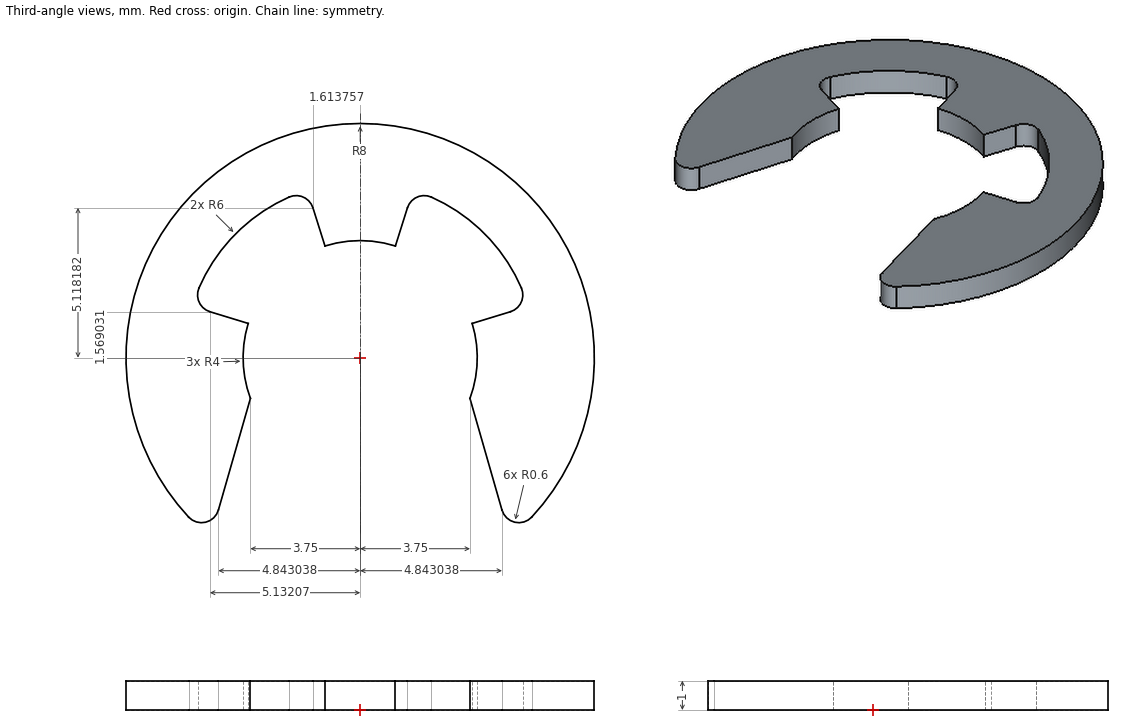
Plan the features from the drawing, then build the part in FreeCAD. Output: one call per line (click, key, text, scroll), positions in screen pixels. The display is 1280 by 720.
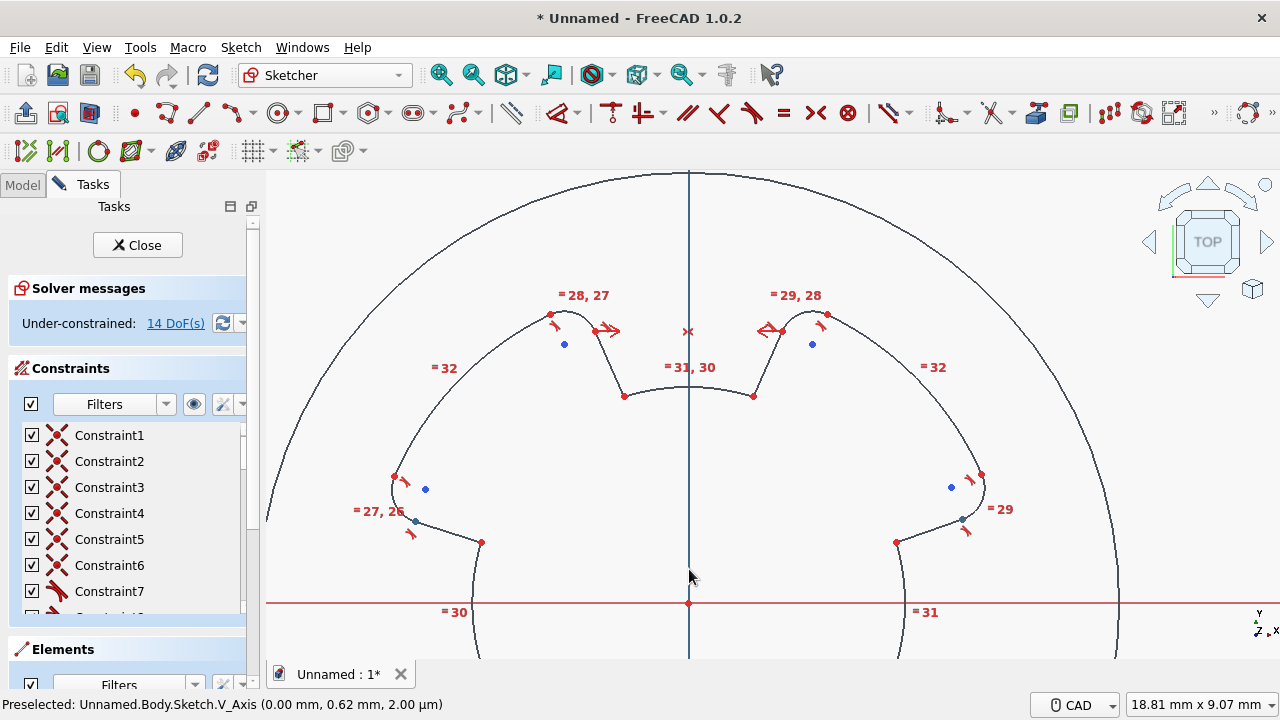
click(816, 114)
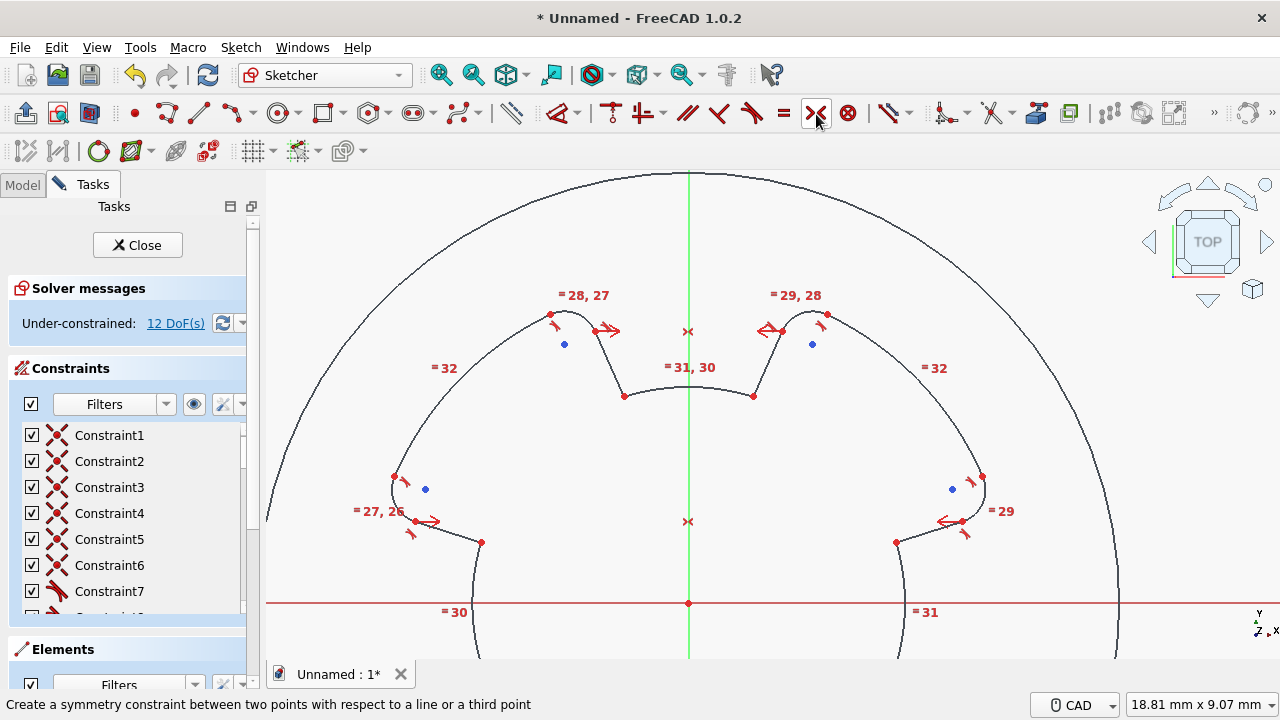
click(558, 114)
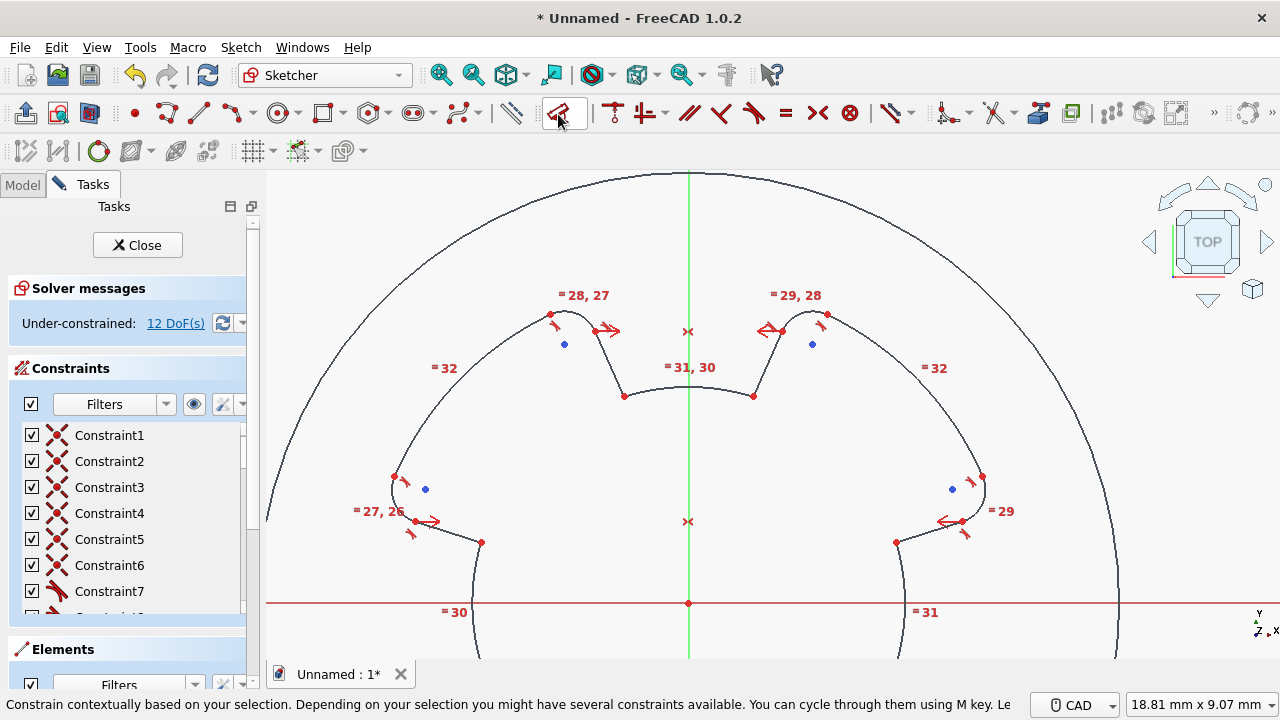
scroll(717, 313, down, 4)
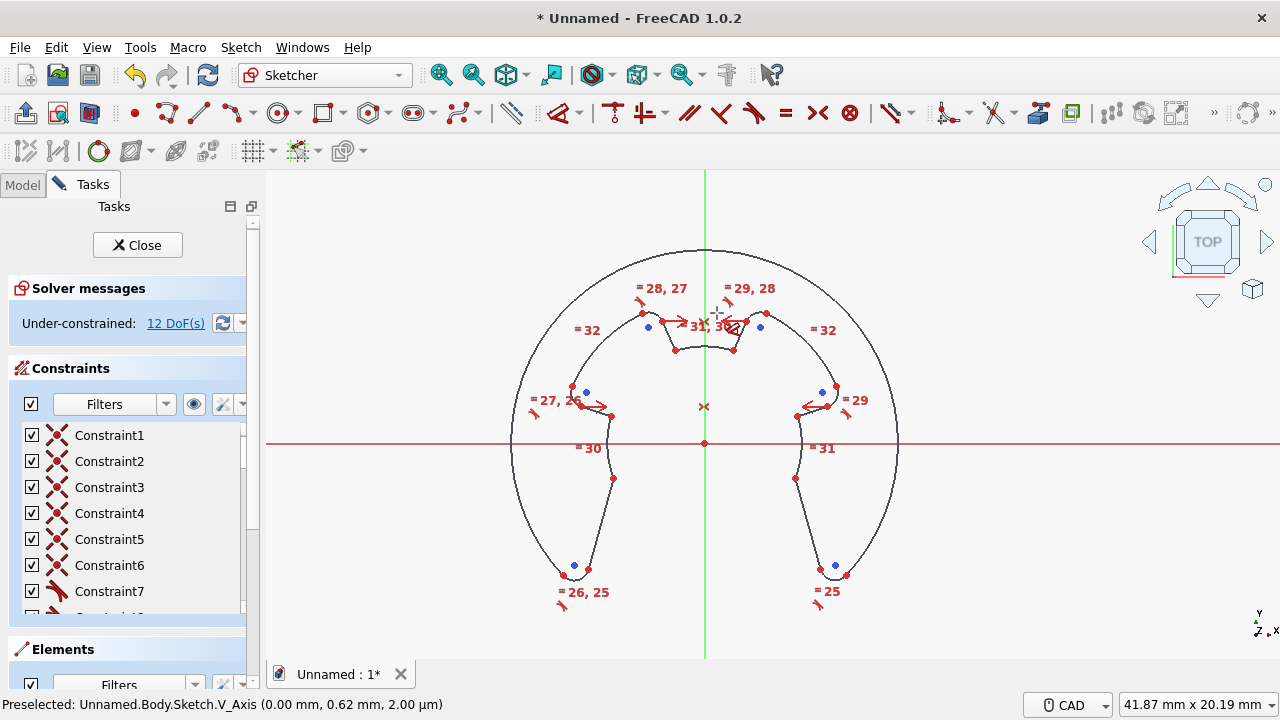
scroll(826, 577, up, 6)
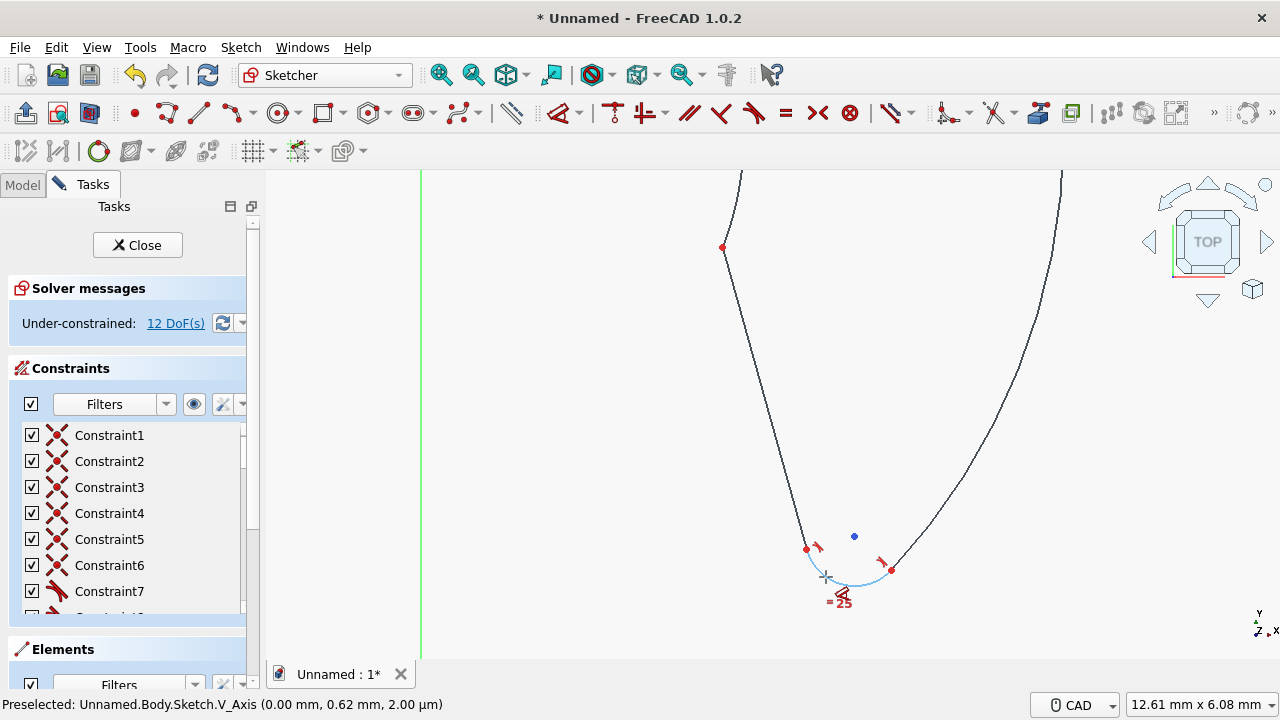
click(824, 576)
click(804, 601)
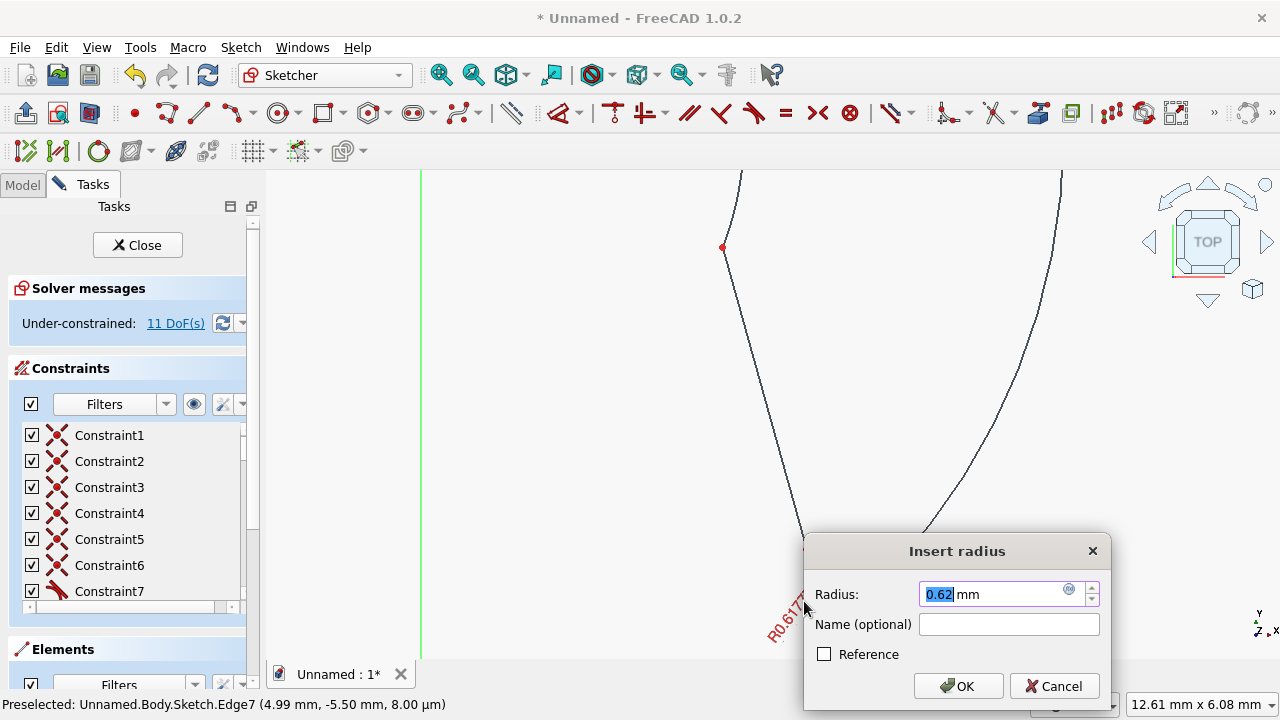
text(0.6)
key(Return)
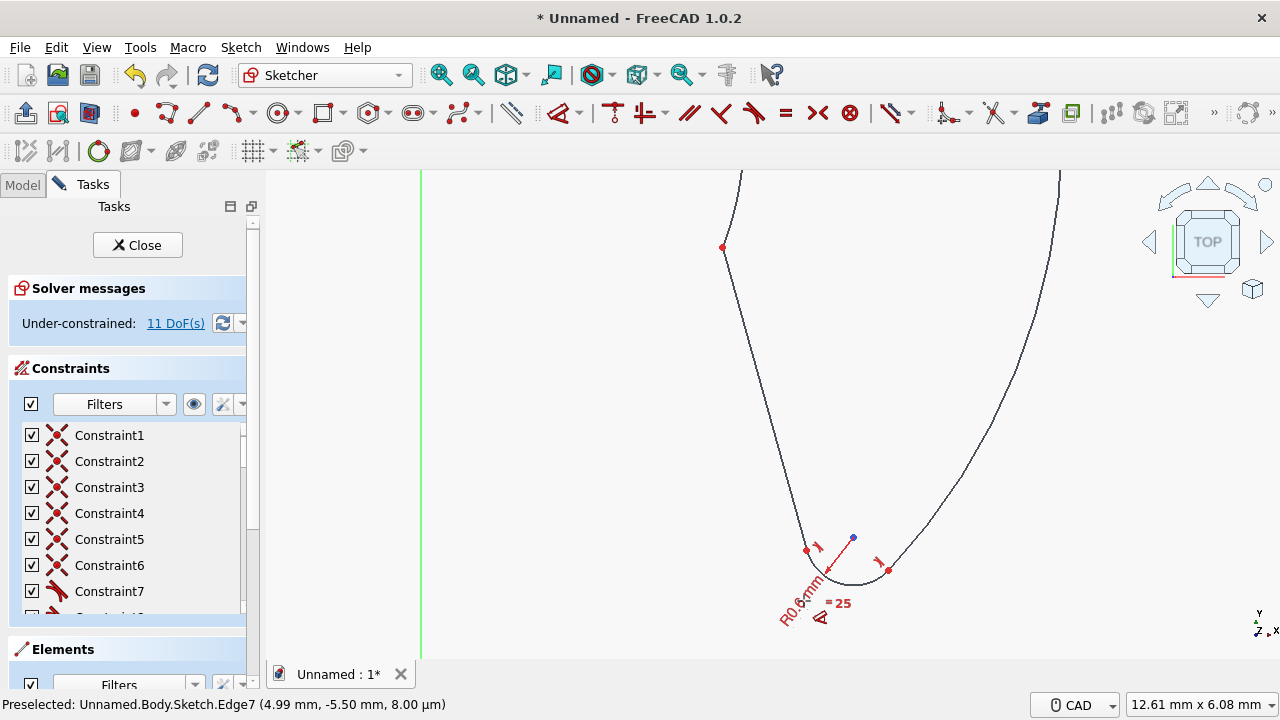
scroll(827, 577, down, 6)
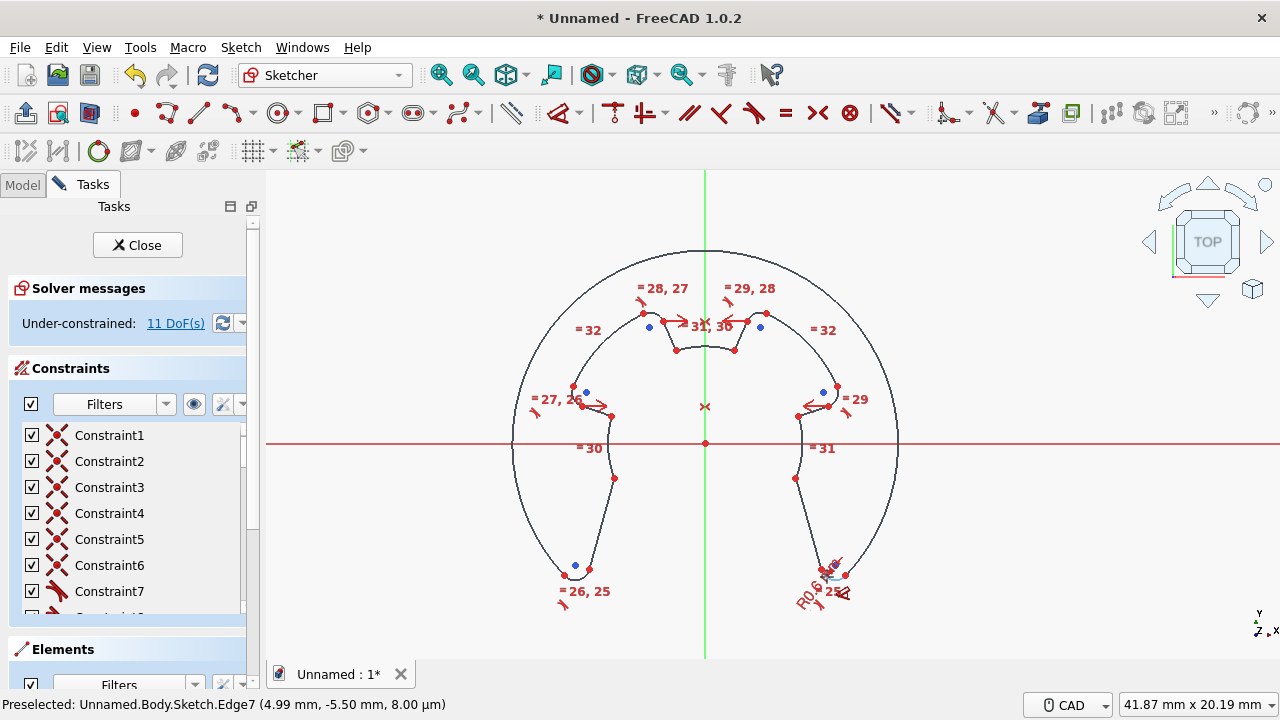
click(860, 328)
click(886, 309)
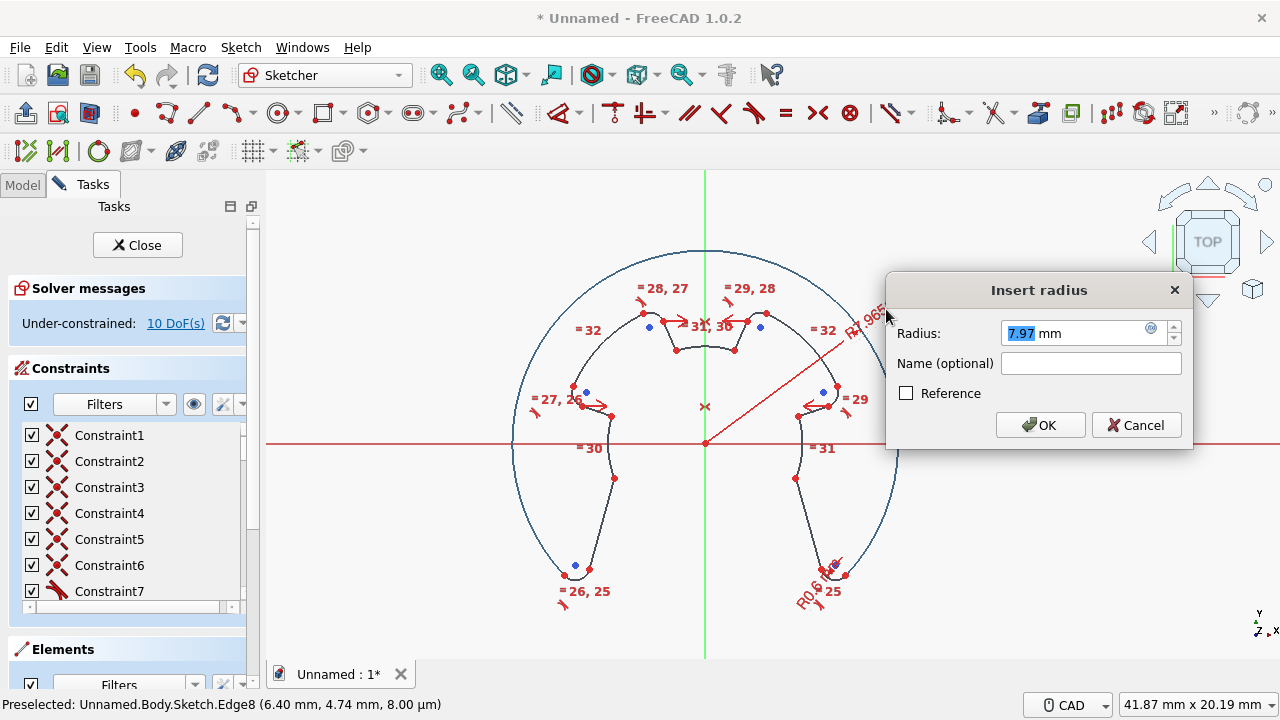
text(8)
key(Return)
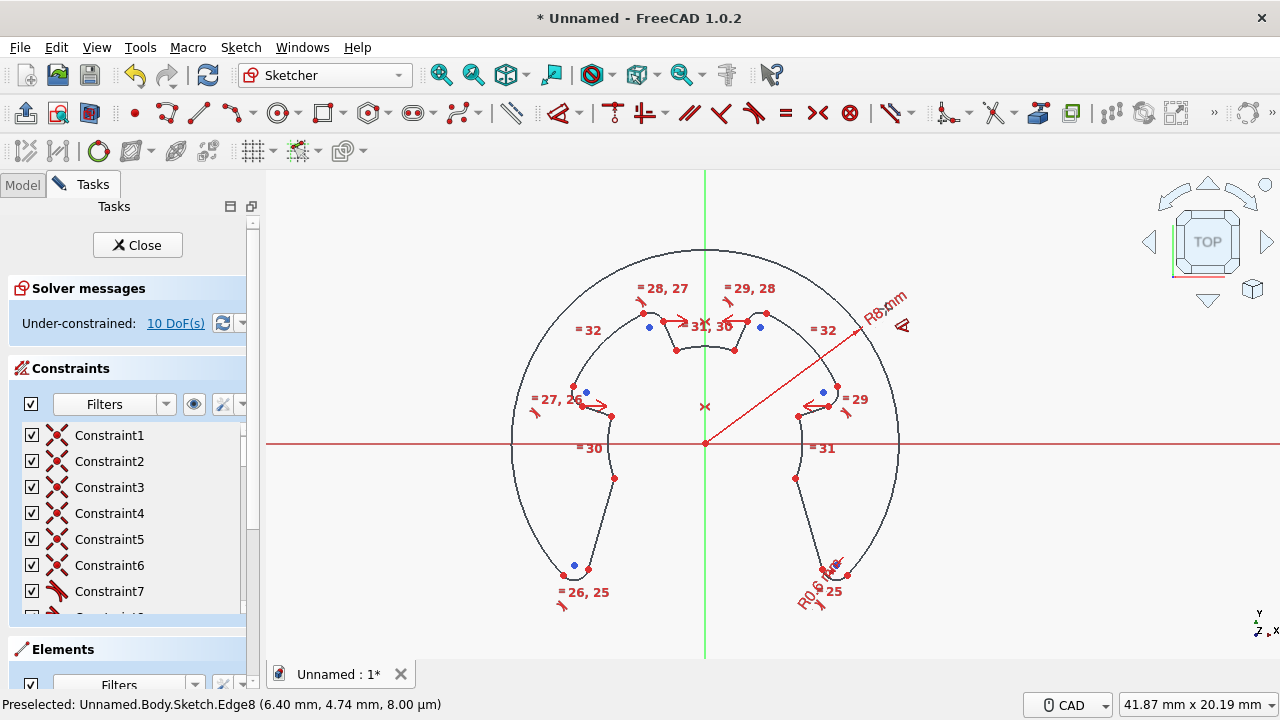
click(609, 460)
click(577, 465)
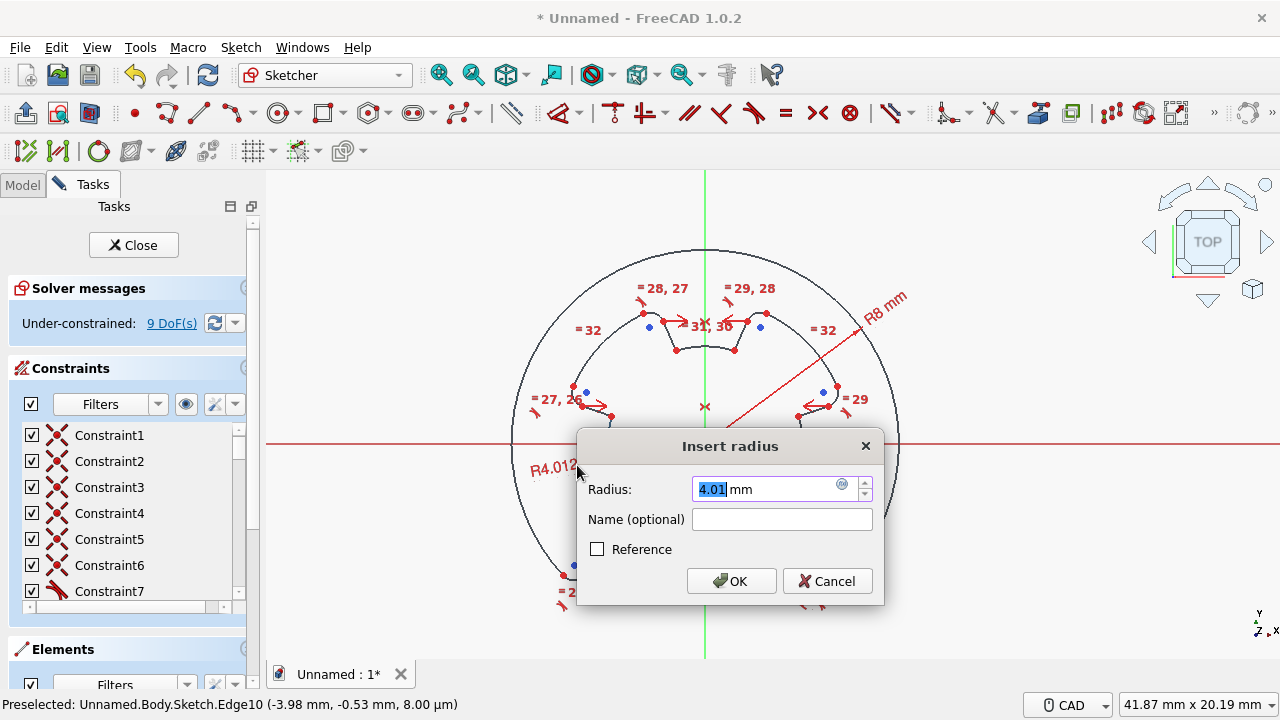
text(4)
key(Return)